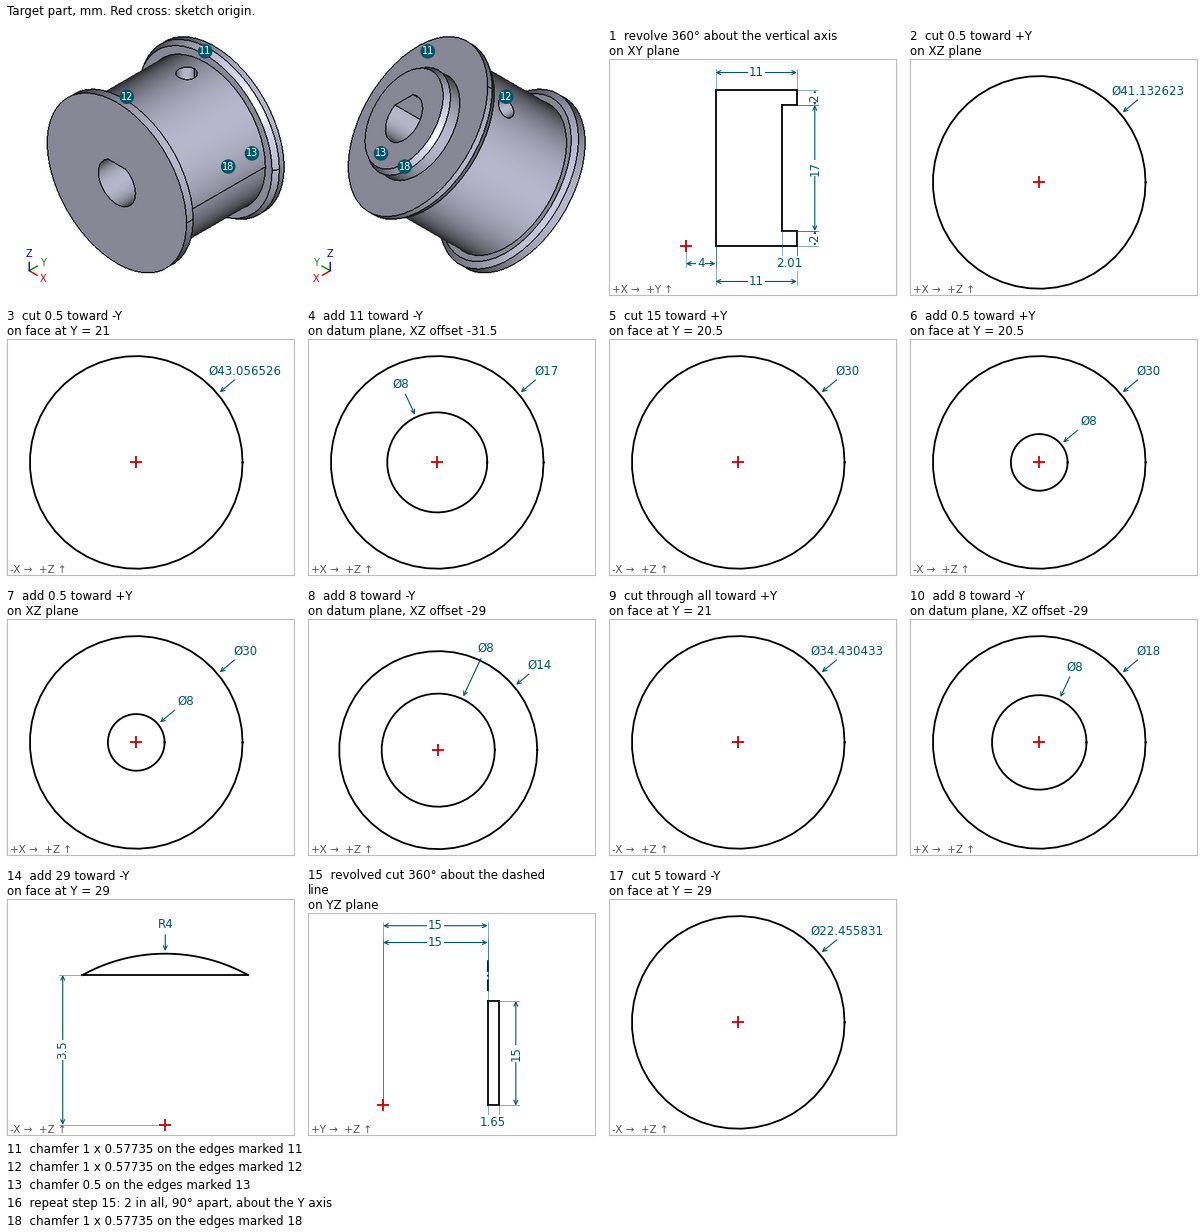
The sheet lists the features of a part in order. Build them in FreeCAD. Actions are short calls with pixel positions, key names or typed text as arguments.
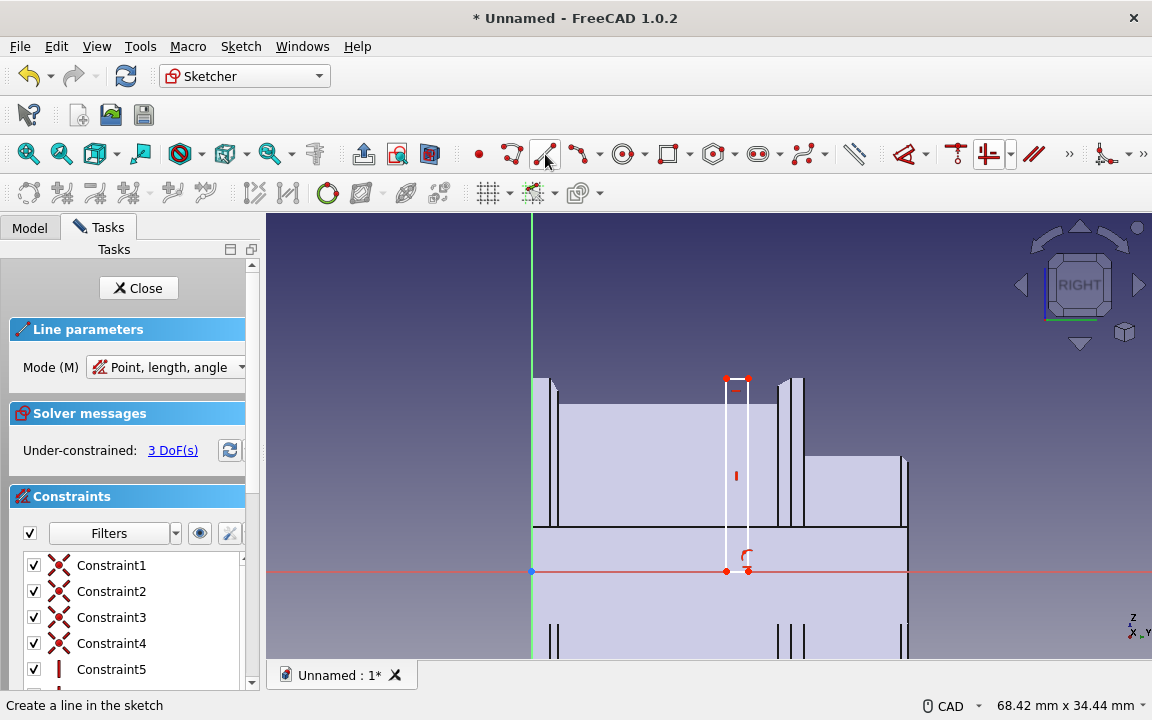
click(726, 358)
click(726, 300)
key(Escape)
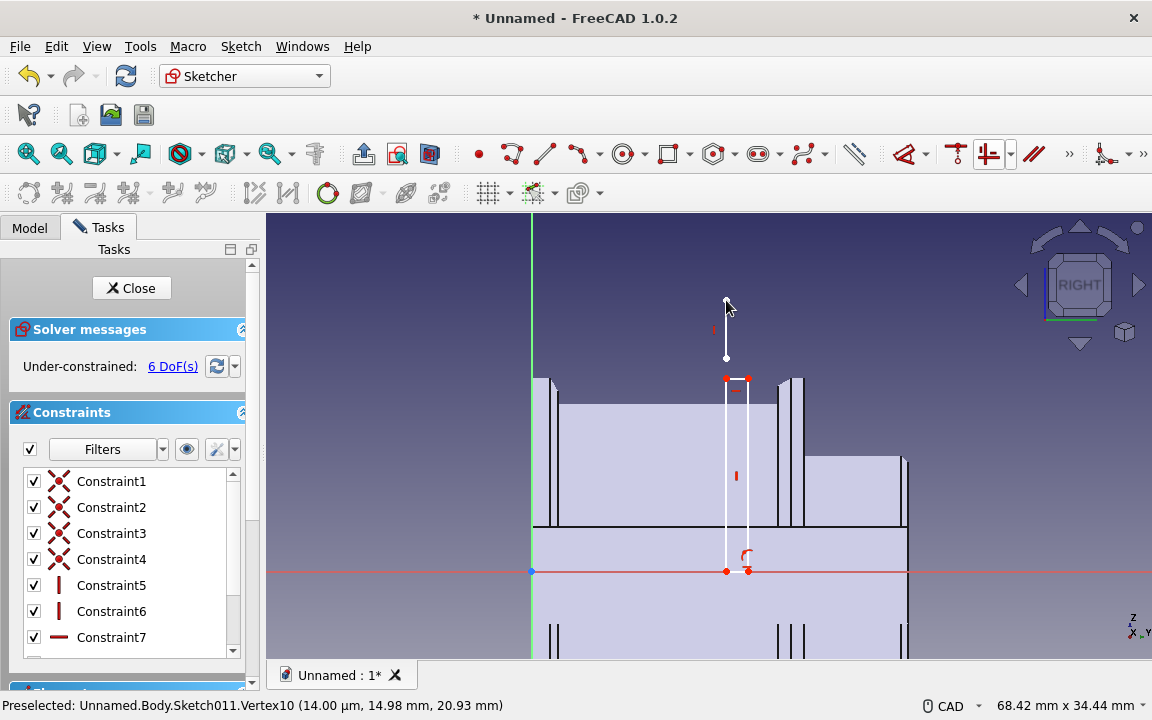
click(726, 342)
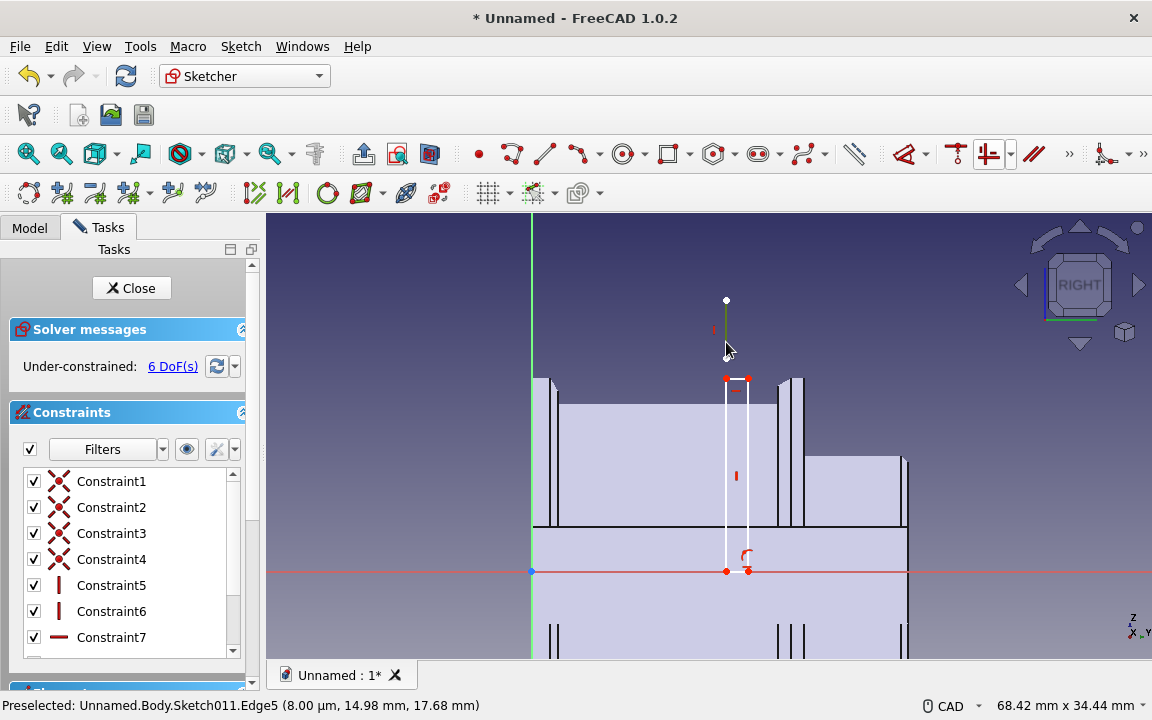
click(855, 154)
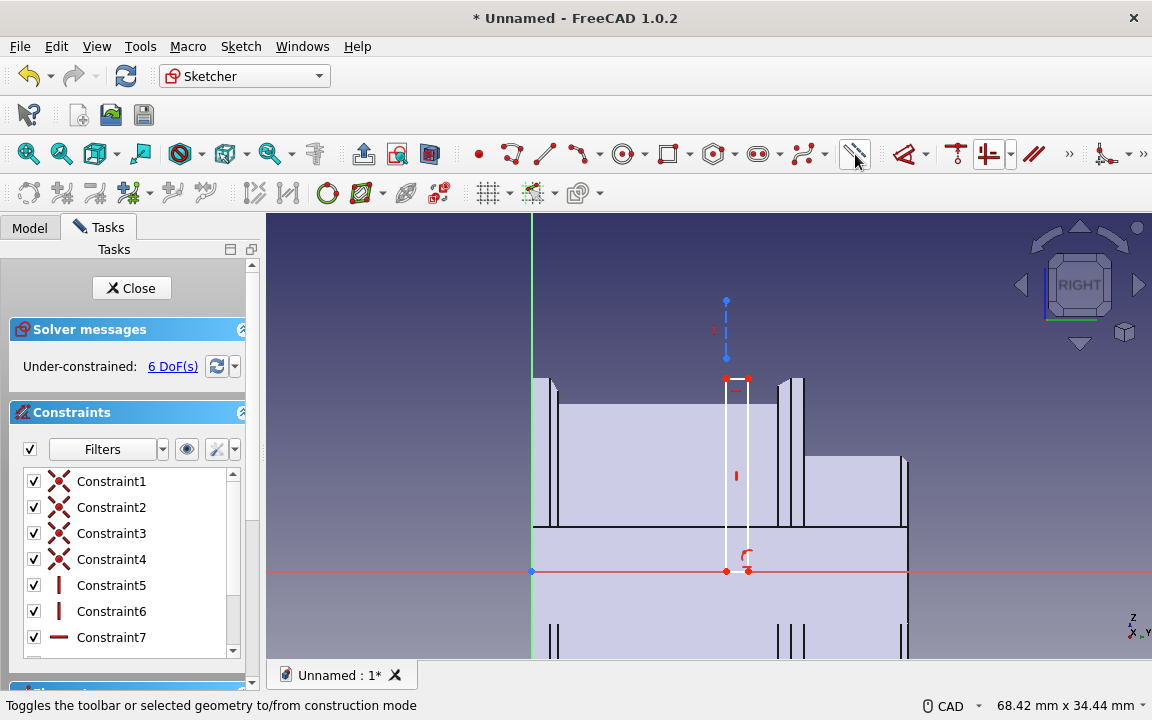
click(904, 154)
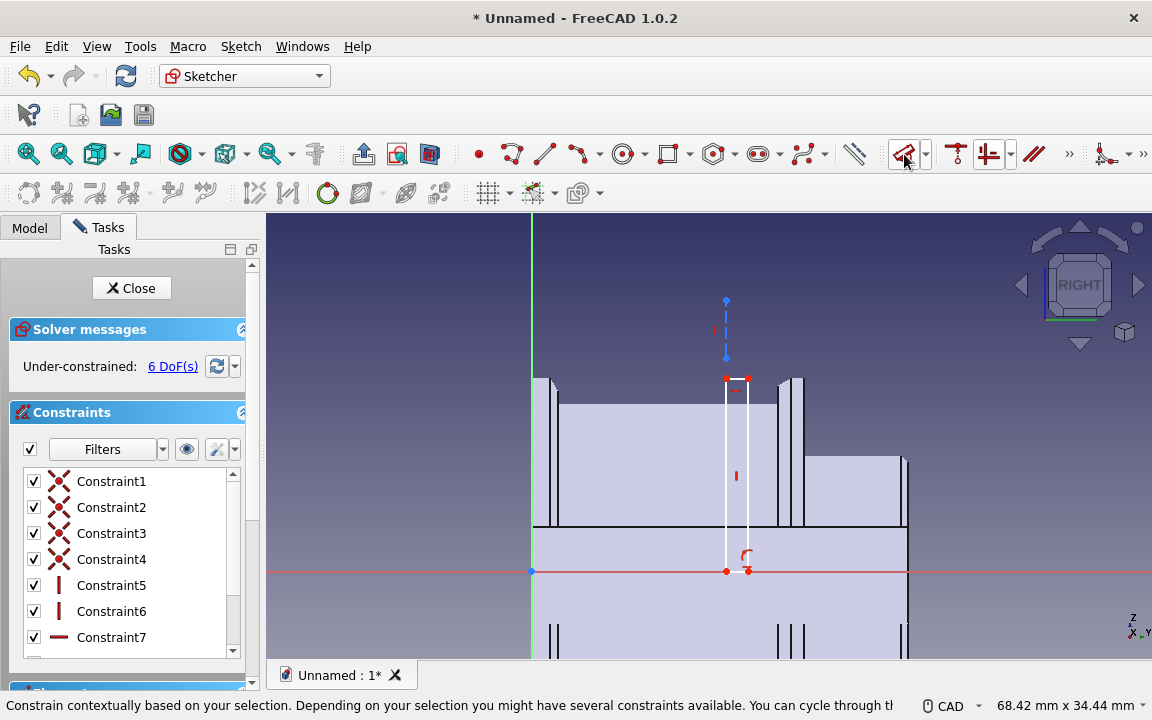
click(726, 437)
click(692, 475)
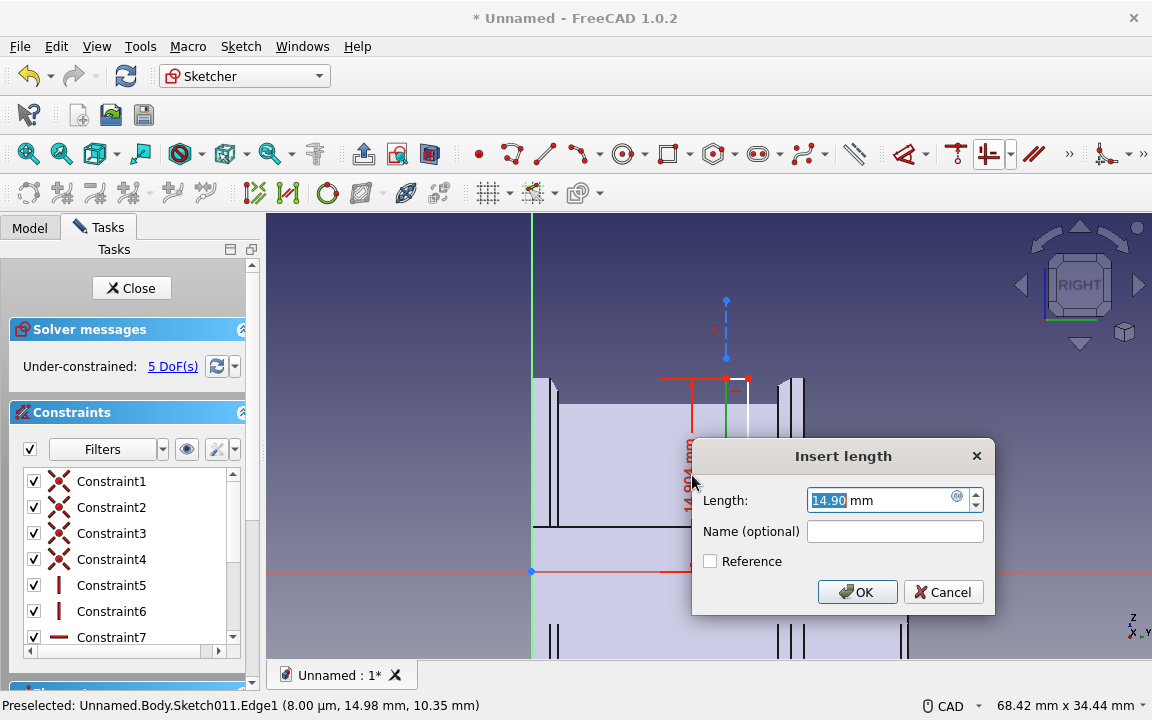
text(15)
key(Return)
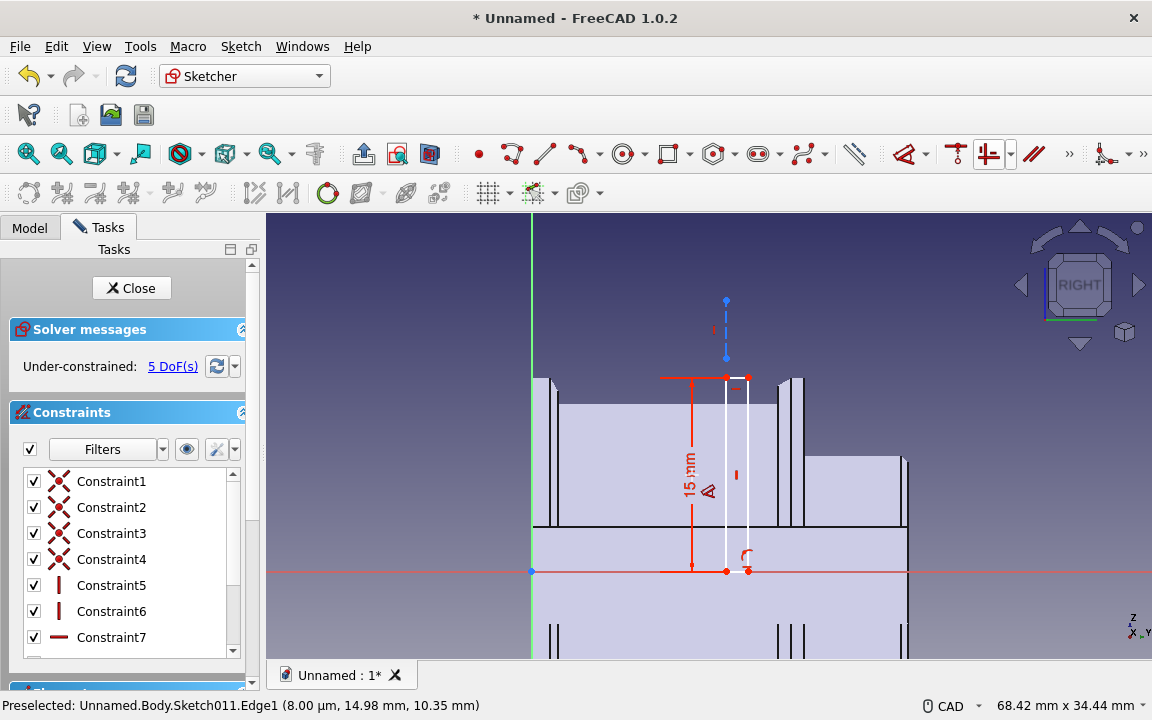
click(726, 378)
click(629, 606)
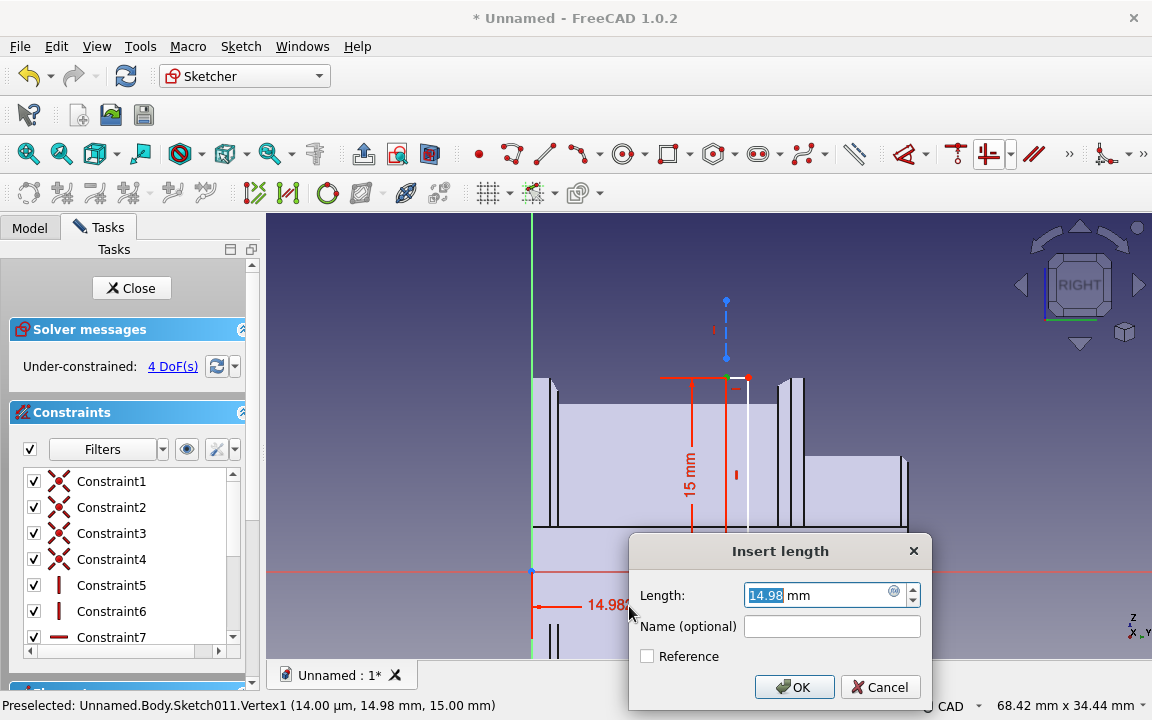
text(15)
key(Return)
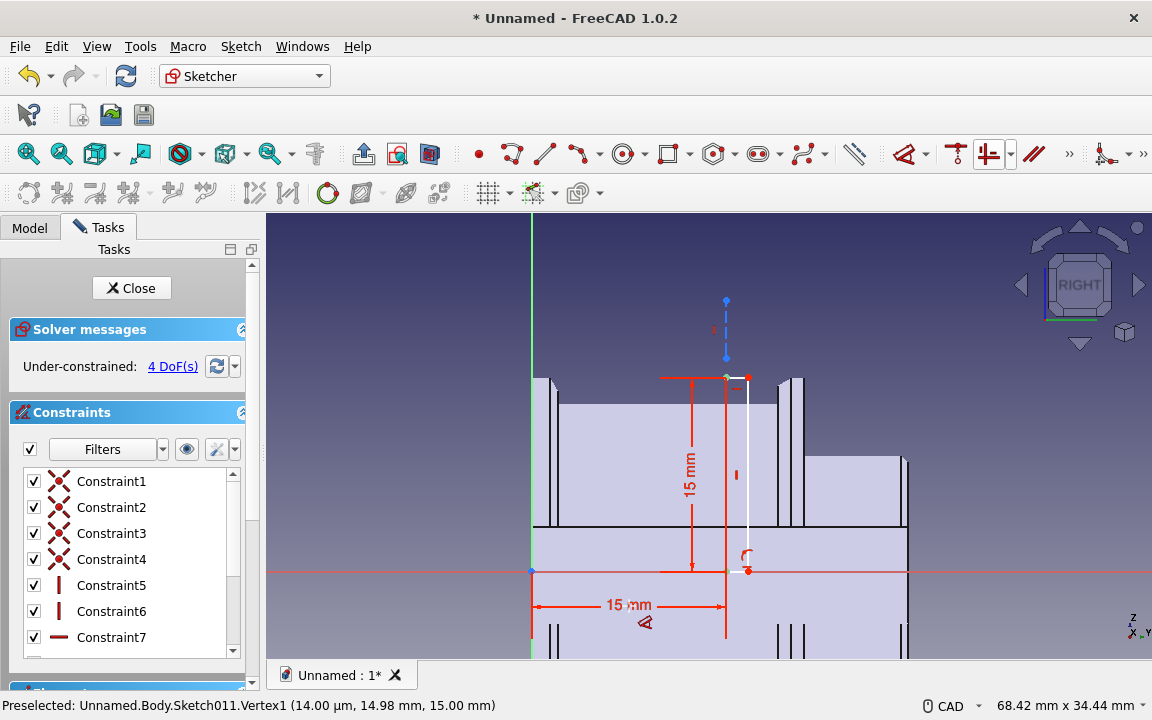
click(726, 359)
click(629, 325)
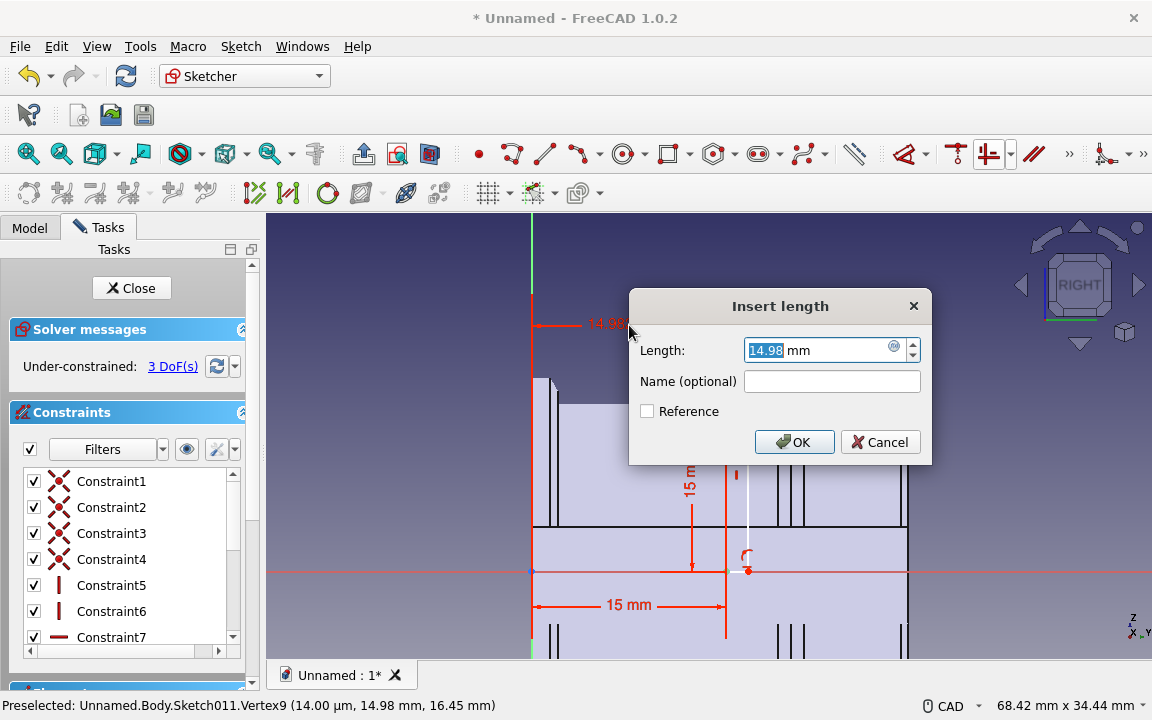
text(15)
key(Return)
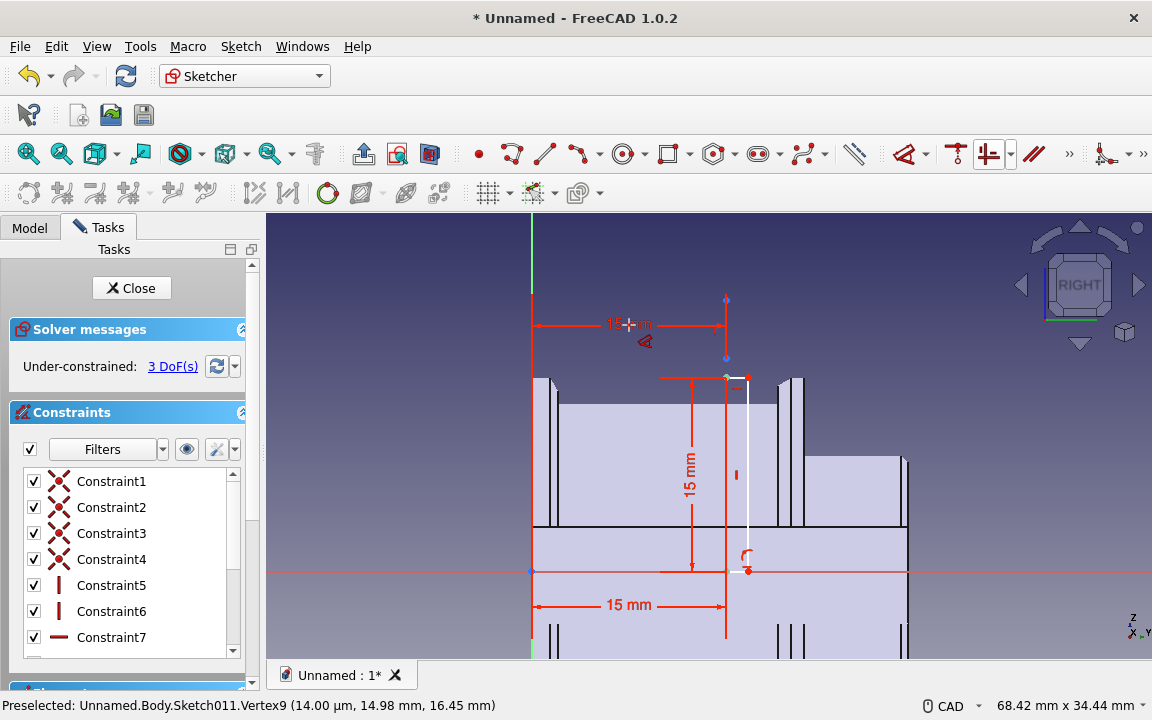
scroll(737, 572, up, 4)